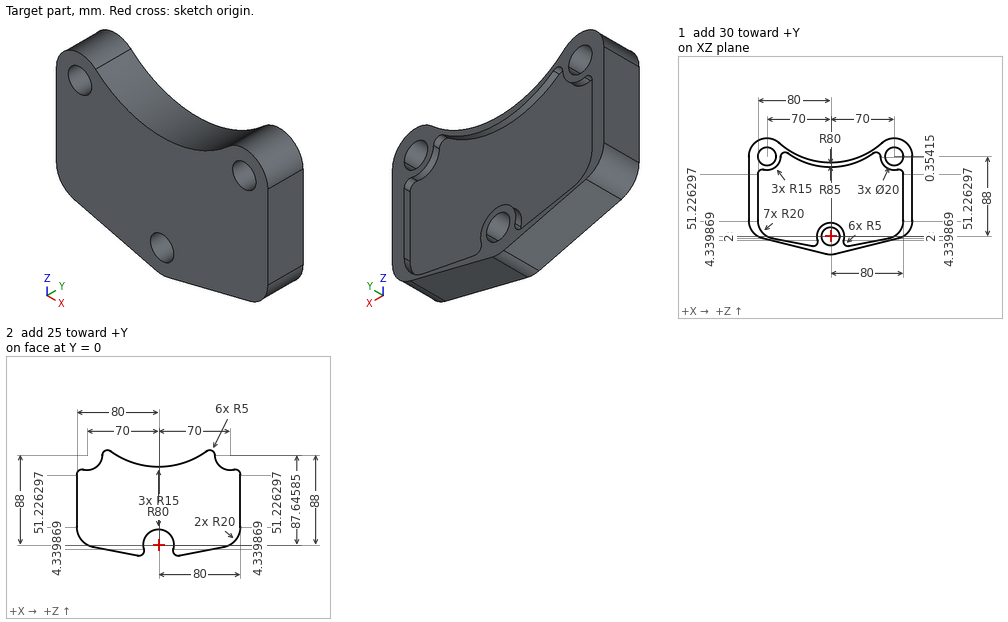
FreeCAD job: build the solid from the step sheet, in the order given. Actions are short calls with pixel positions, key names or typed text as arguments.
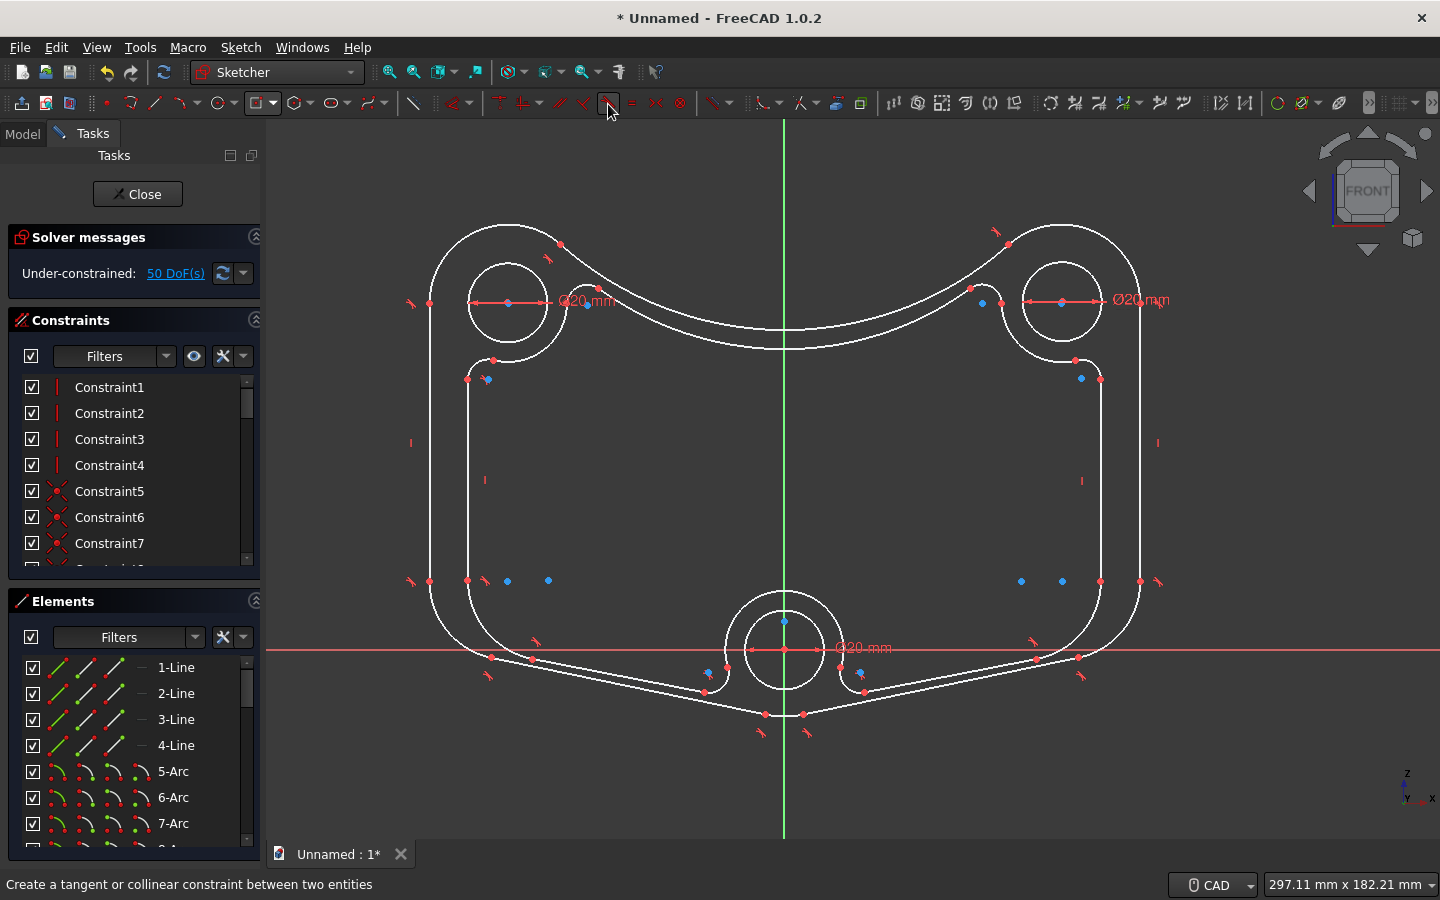
click(1101, 521)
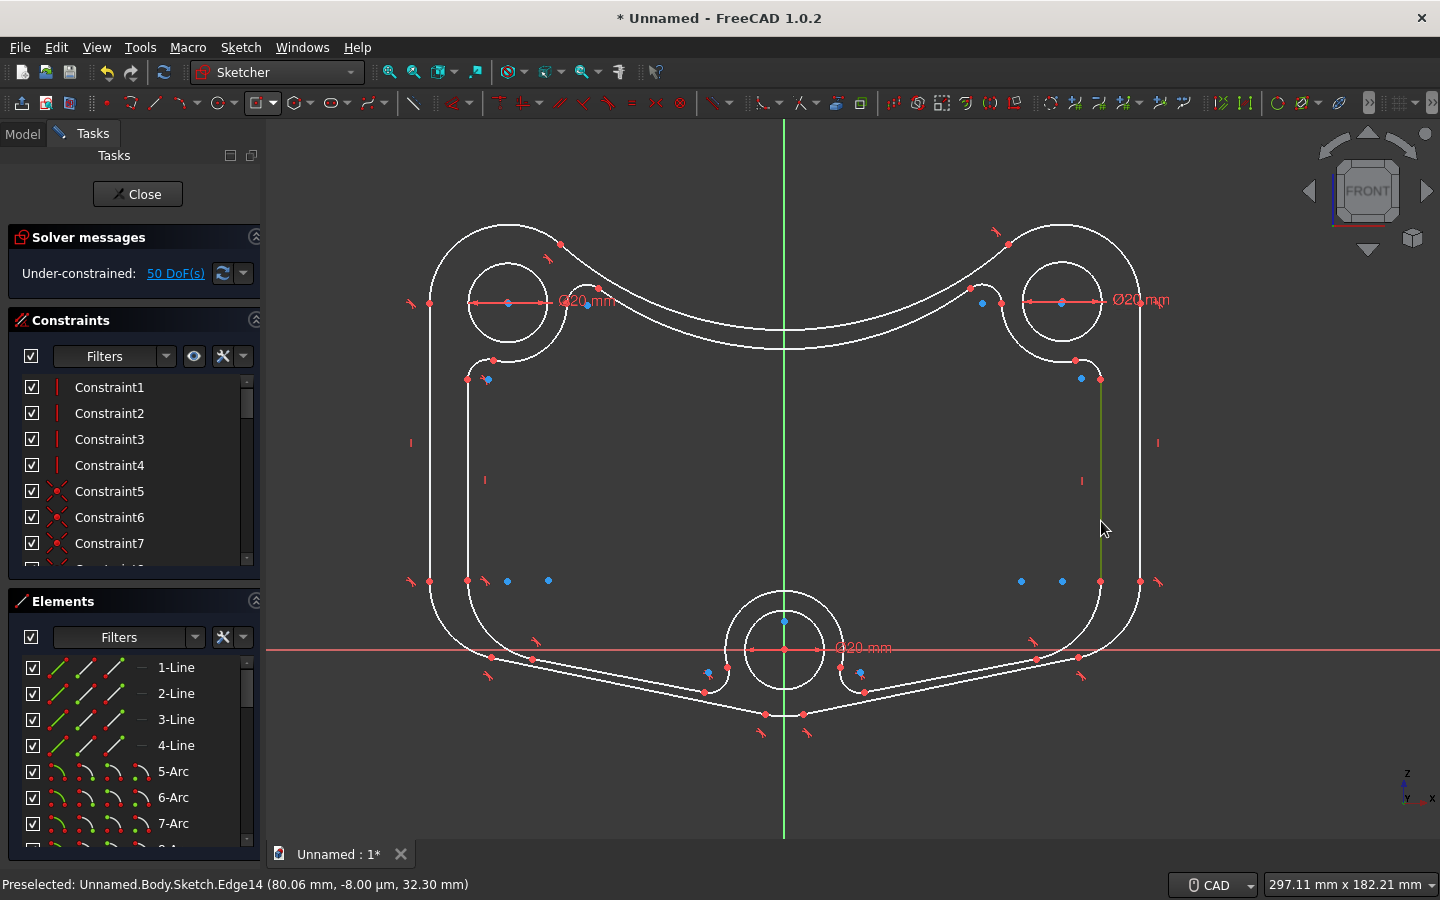
click(1067, 646)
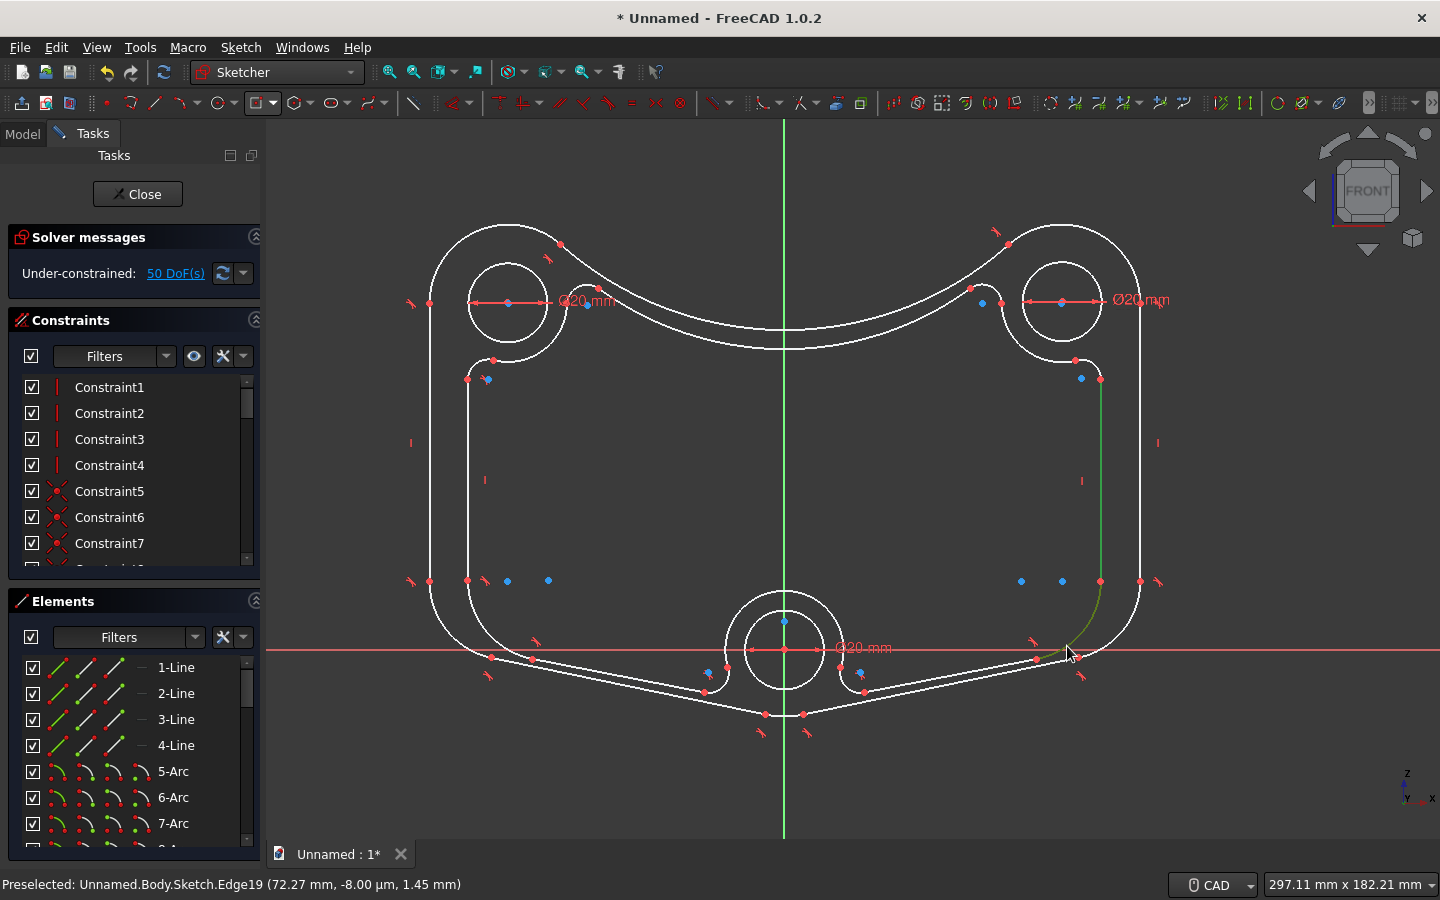
click(608, 104)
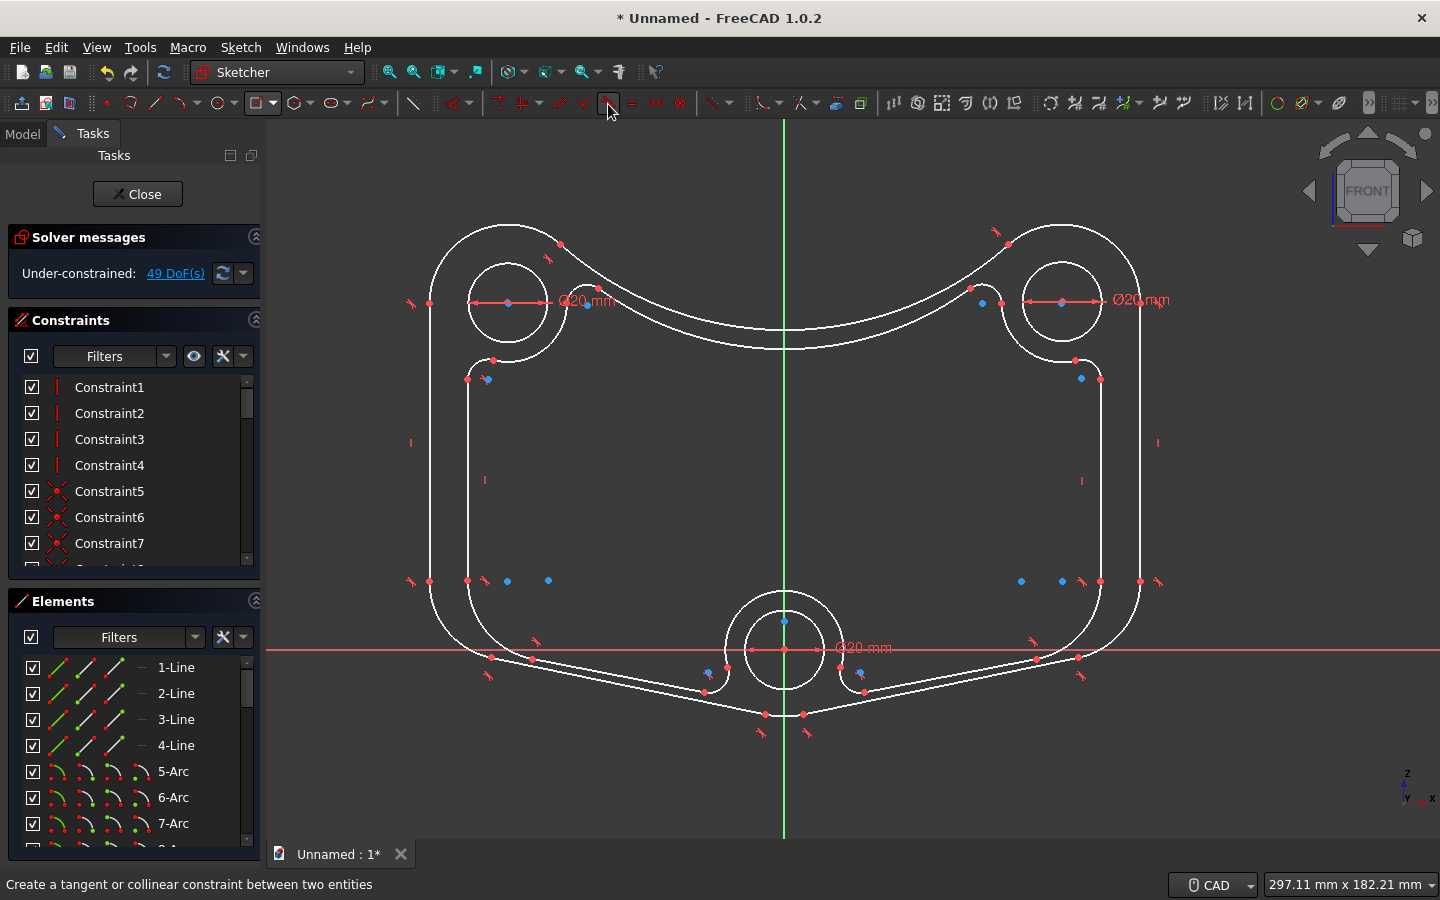
click(1101, 521)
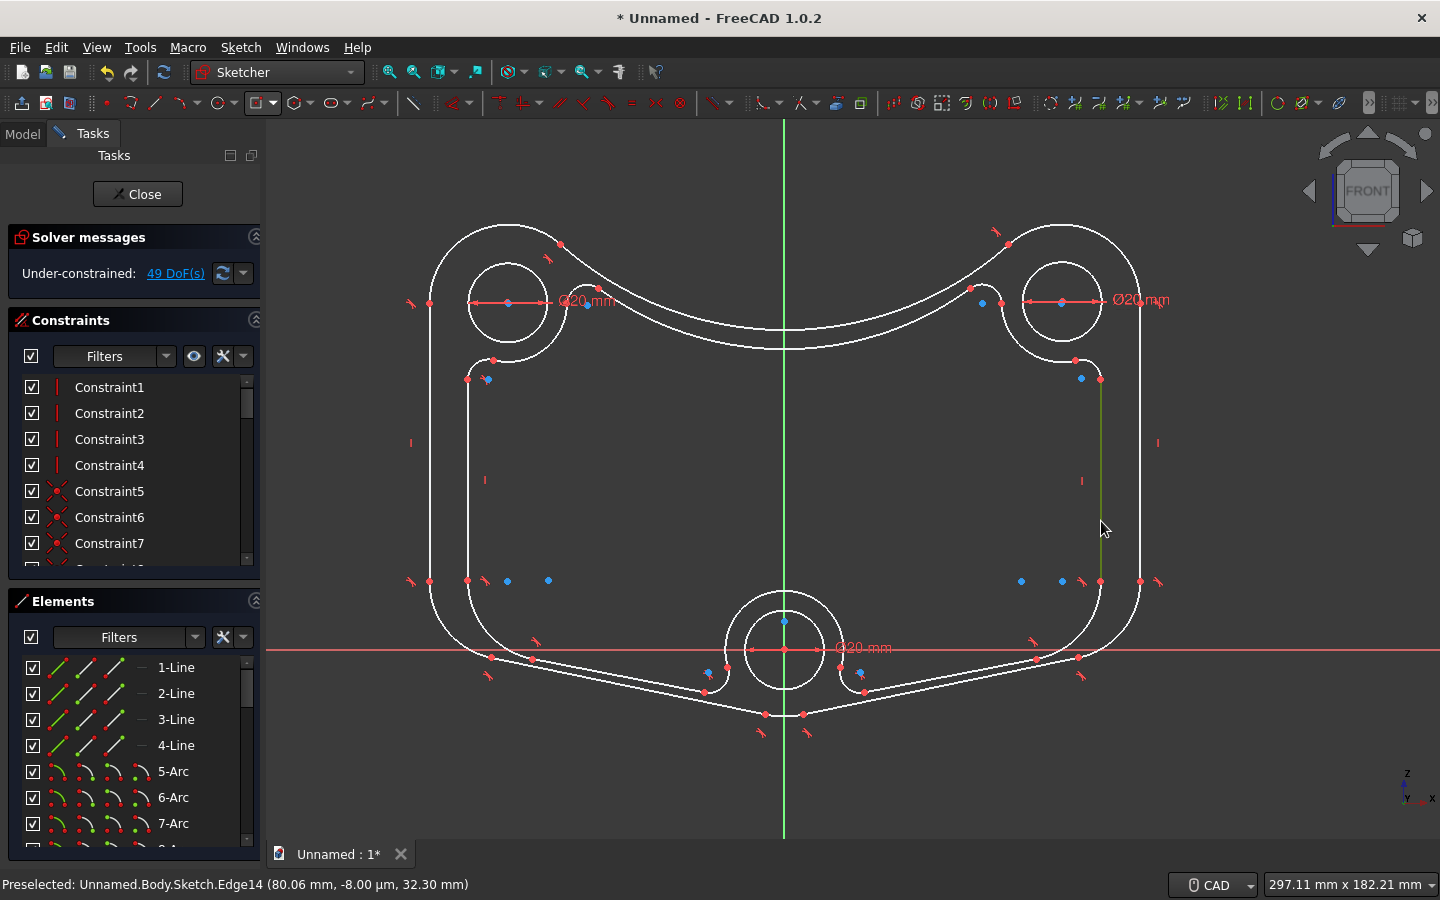
scroll(1098, 369, up, 2)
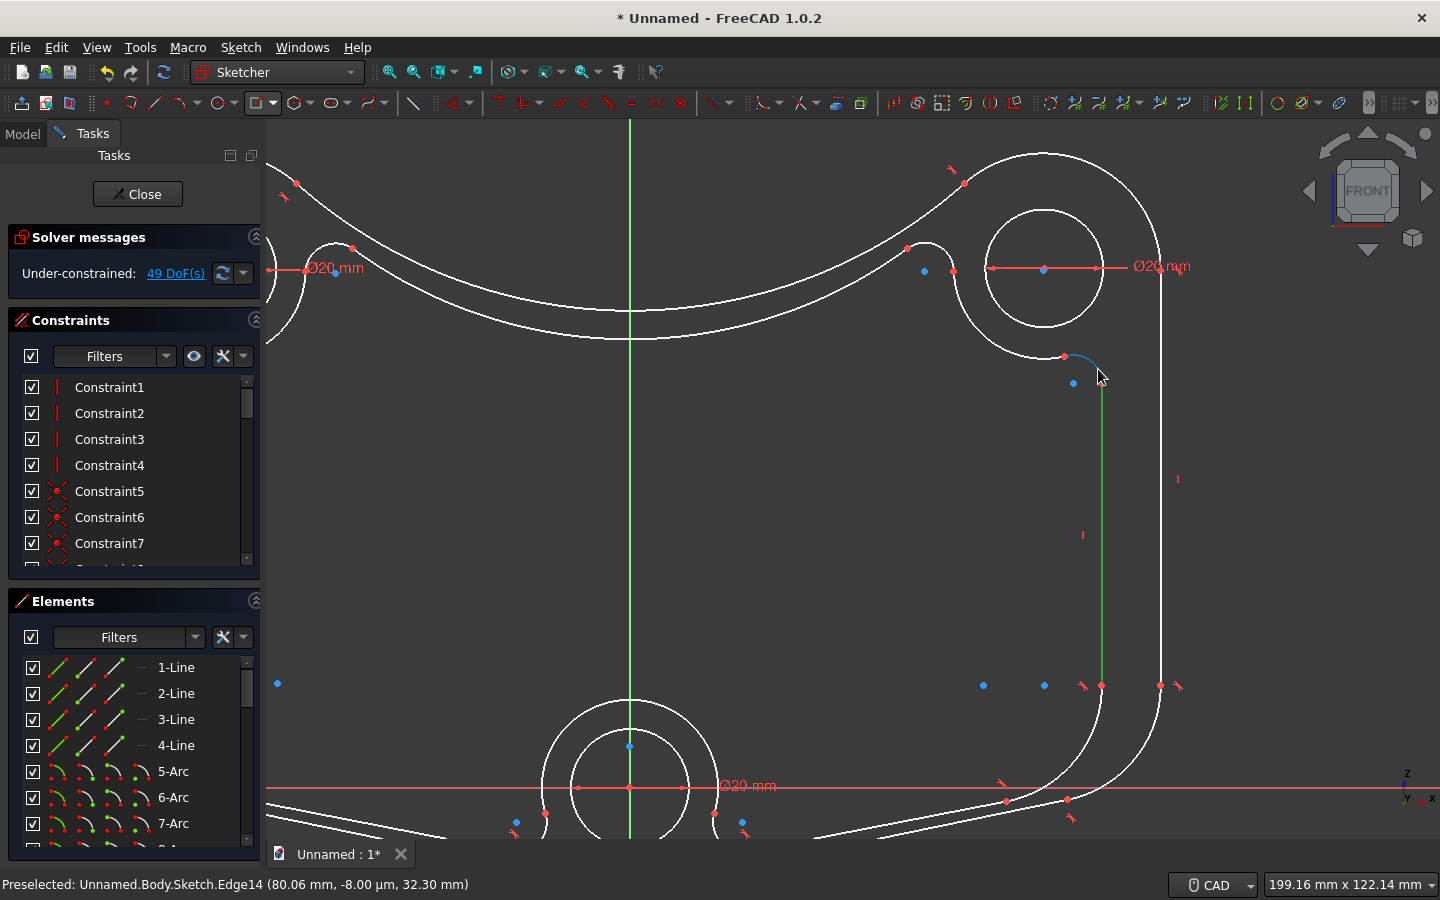
click(1098, 369)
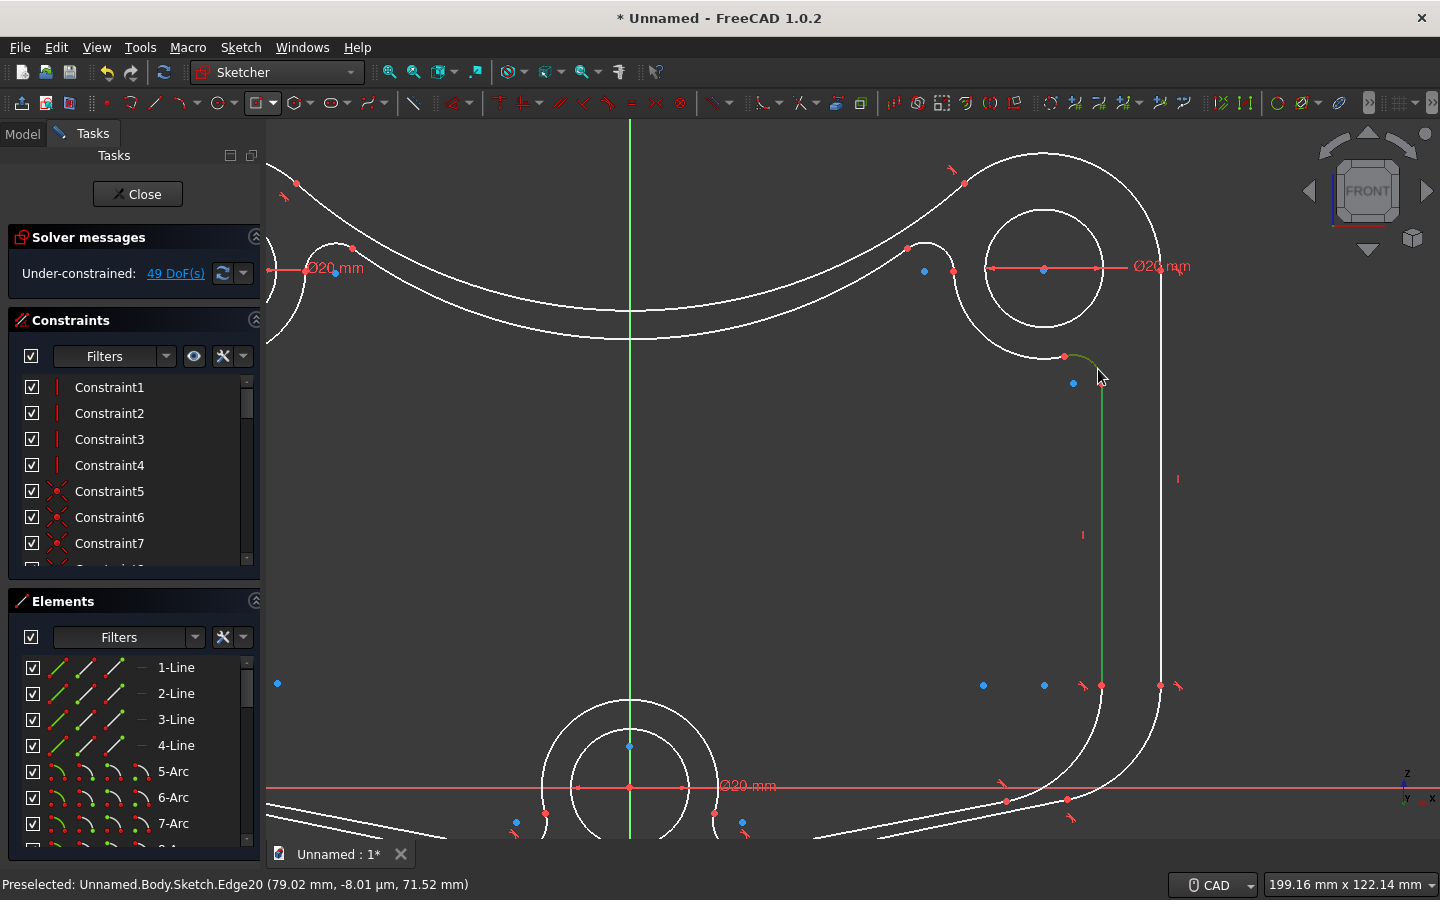
click(608, 104)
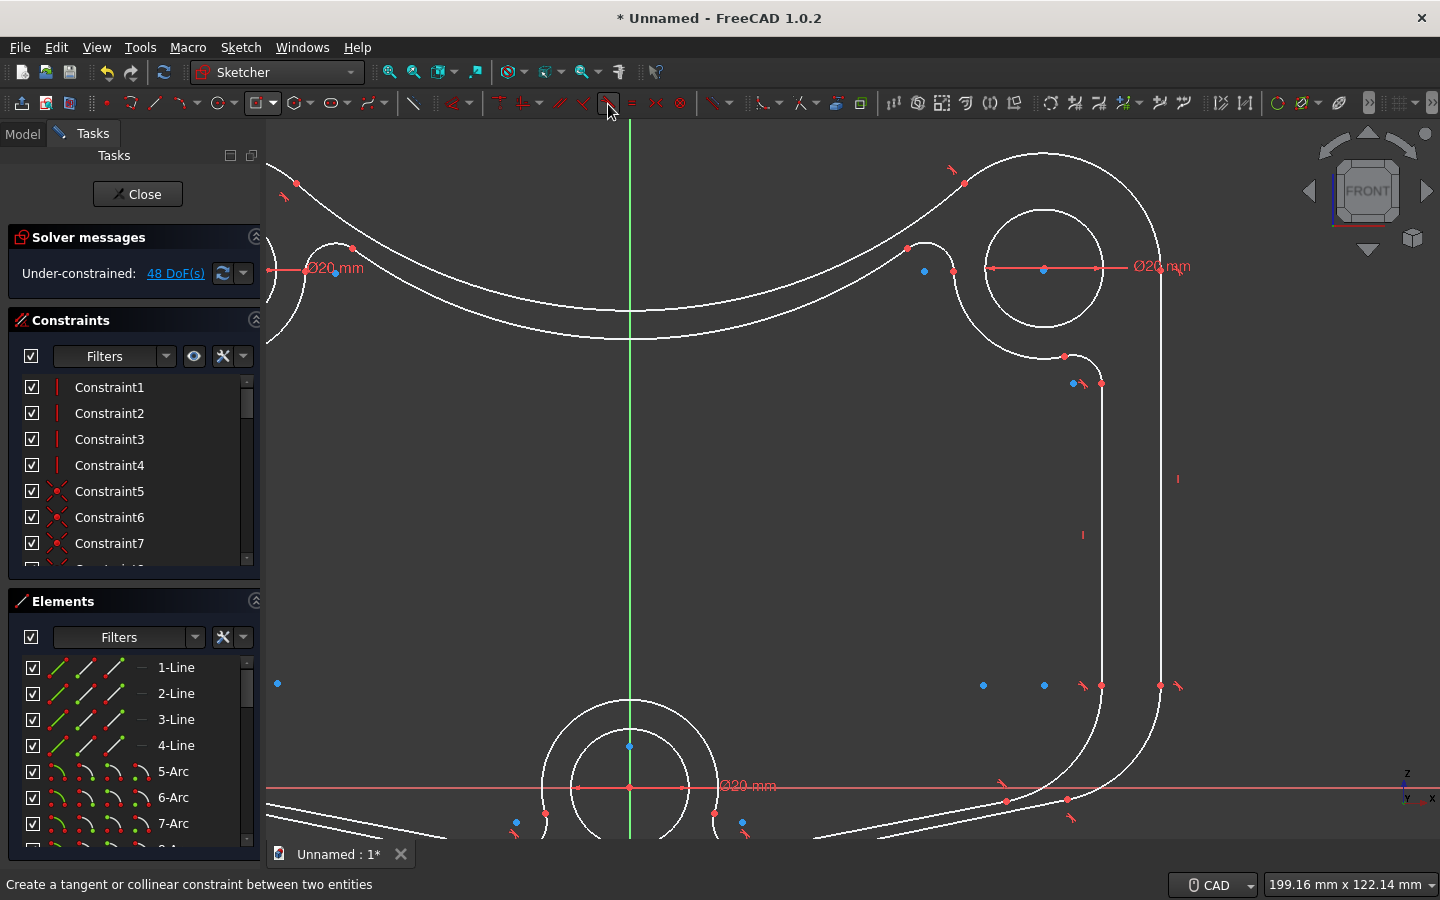
scroll(1099, 369, down, 2)